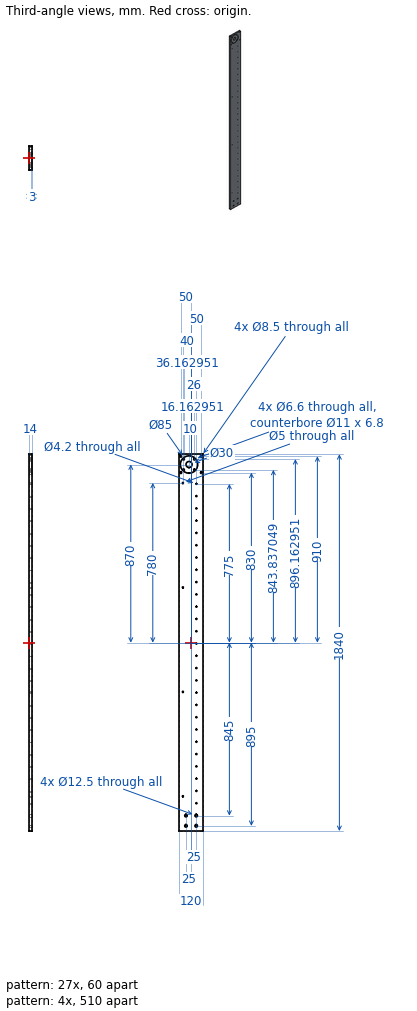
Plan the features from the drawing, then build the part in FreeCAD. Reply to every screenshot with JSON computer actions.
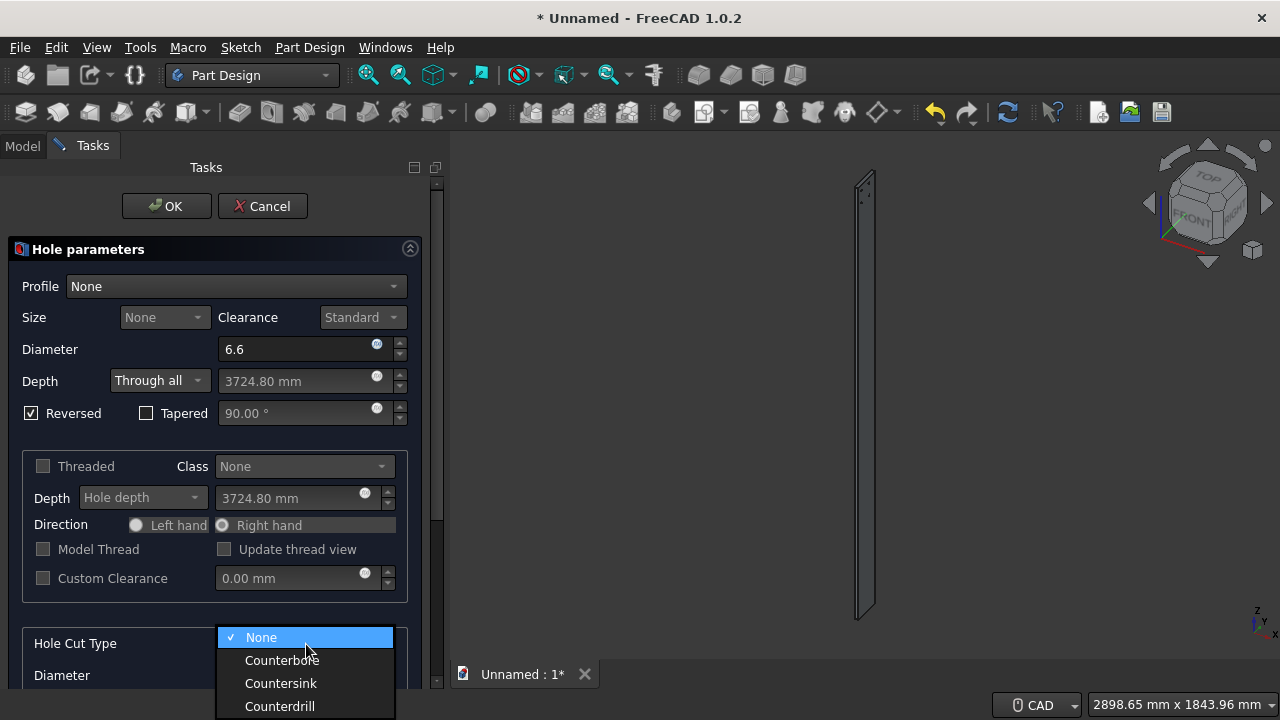
{"action": "left_click", "coordinate": [304, 660]}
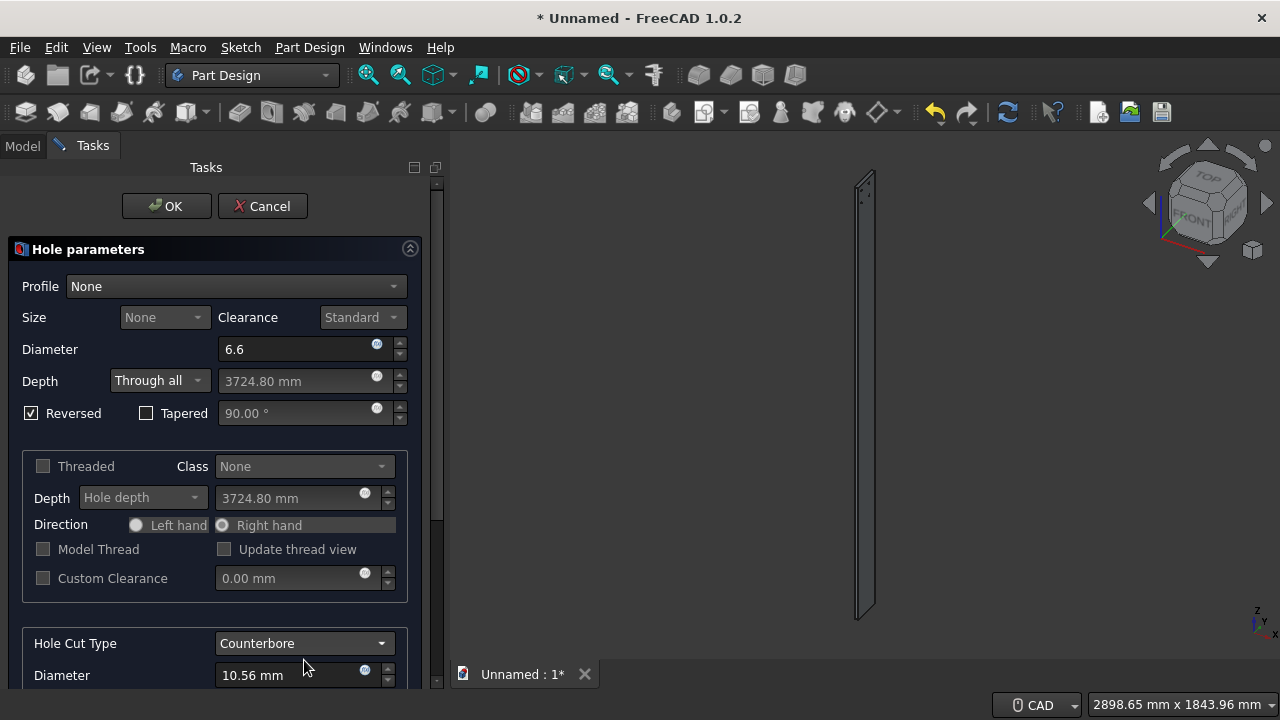
{"action": "triple_click", "coordinate": [298, 675]}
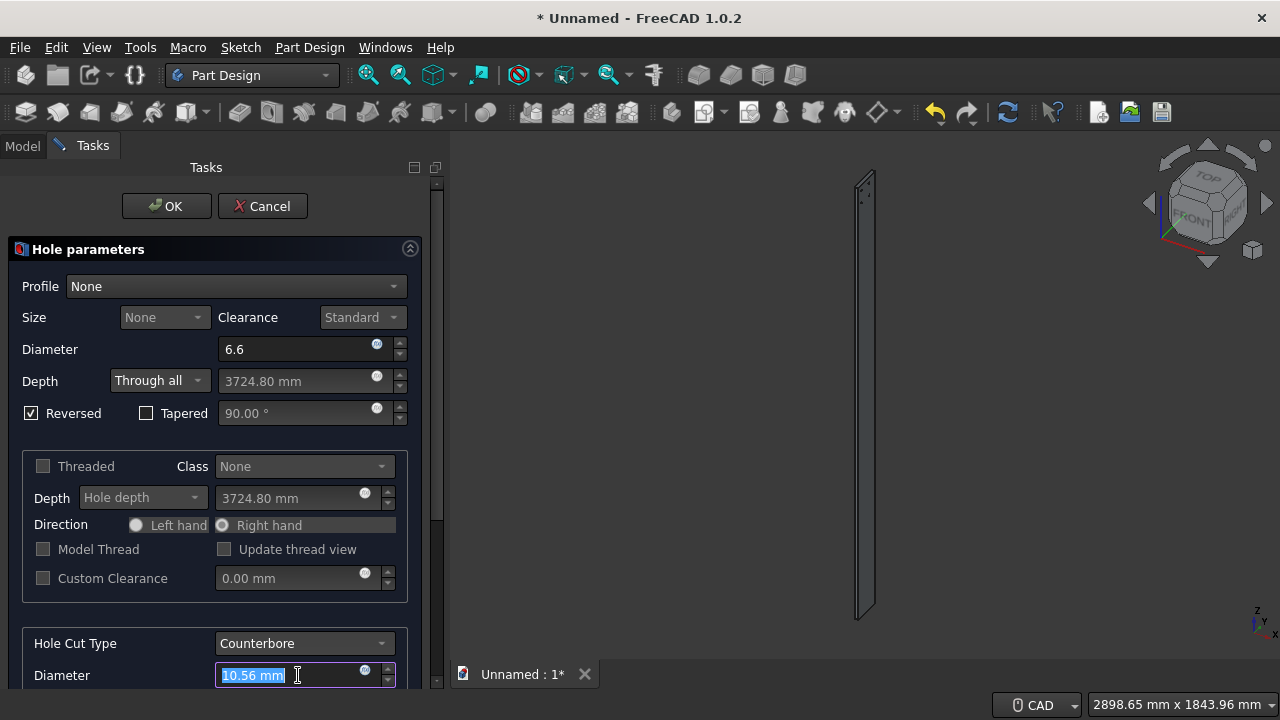
{"action": "type", "text": "11"}
{"action": "key", "text": "Tab"}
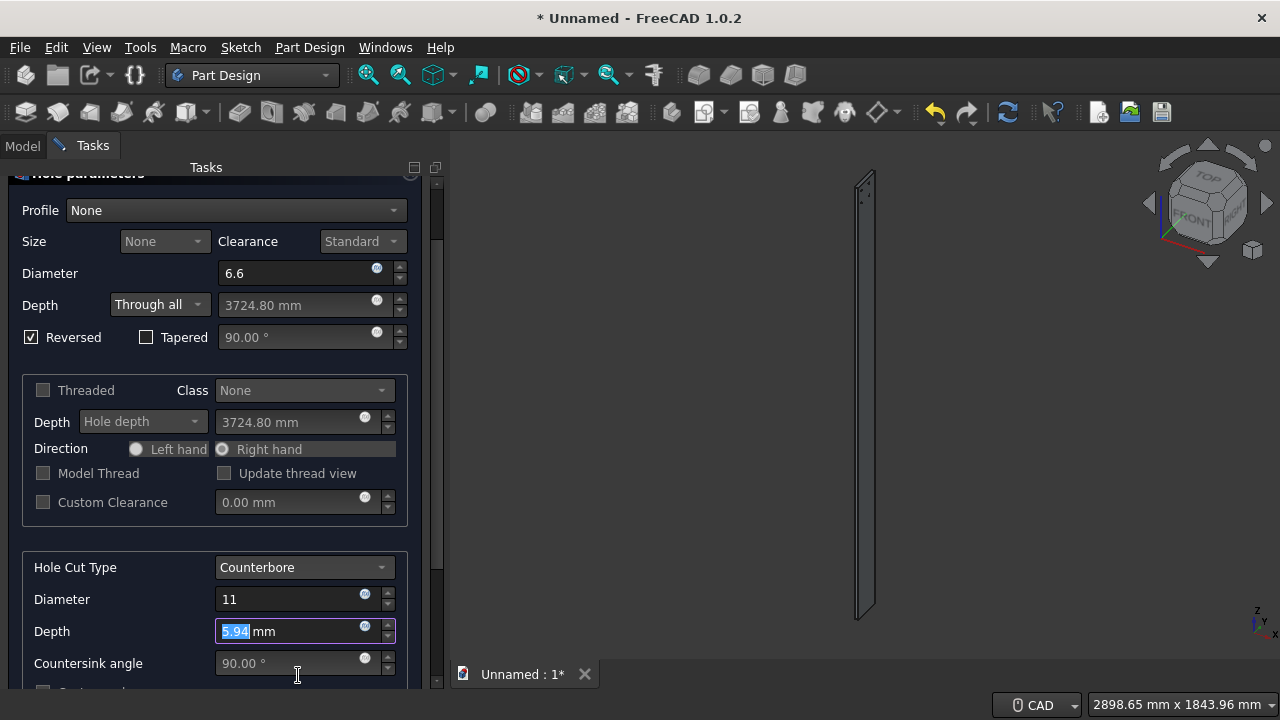
{"action": "type", "text": "6.8"}
{"action": "key", "text": "Tab"}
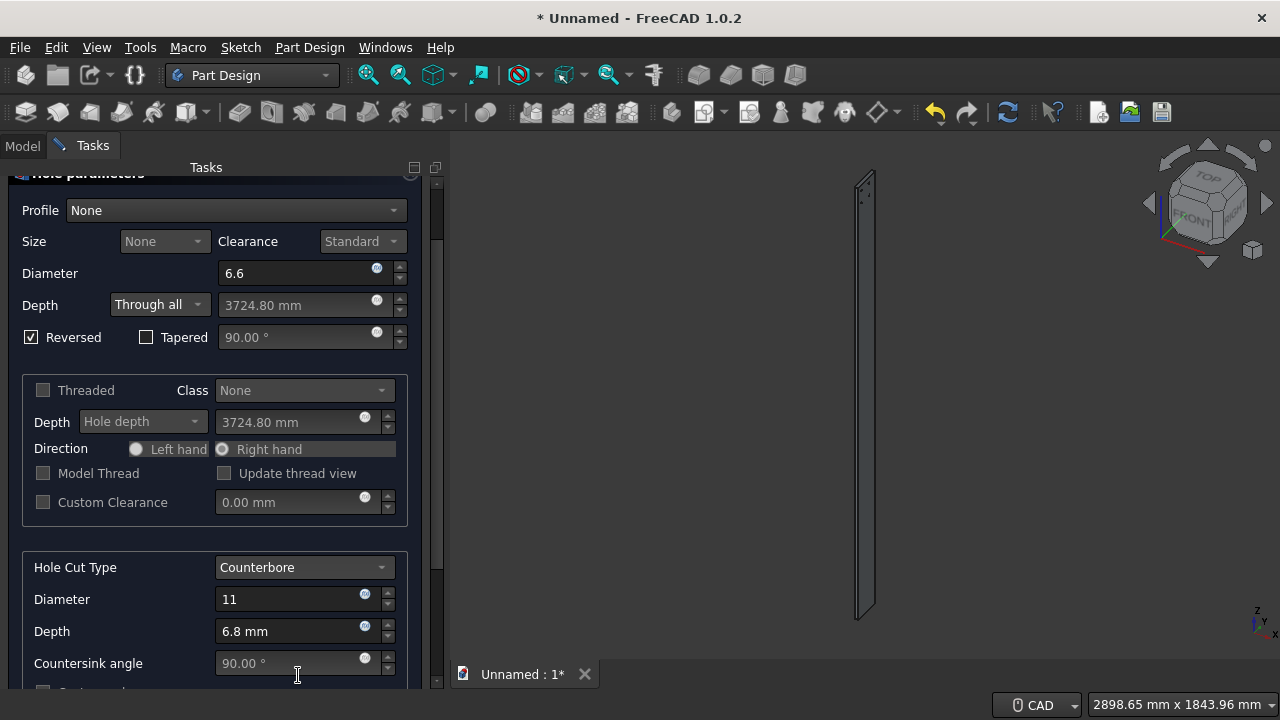
{"action": "scroll", "coordinate": [437, 432], "scroll_direction": "up", "scroll_amount": 3}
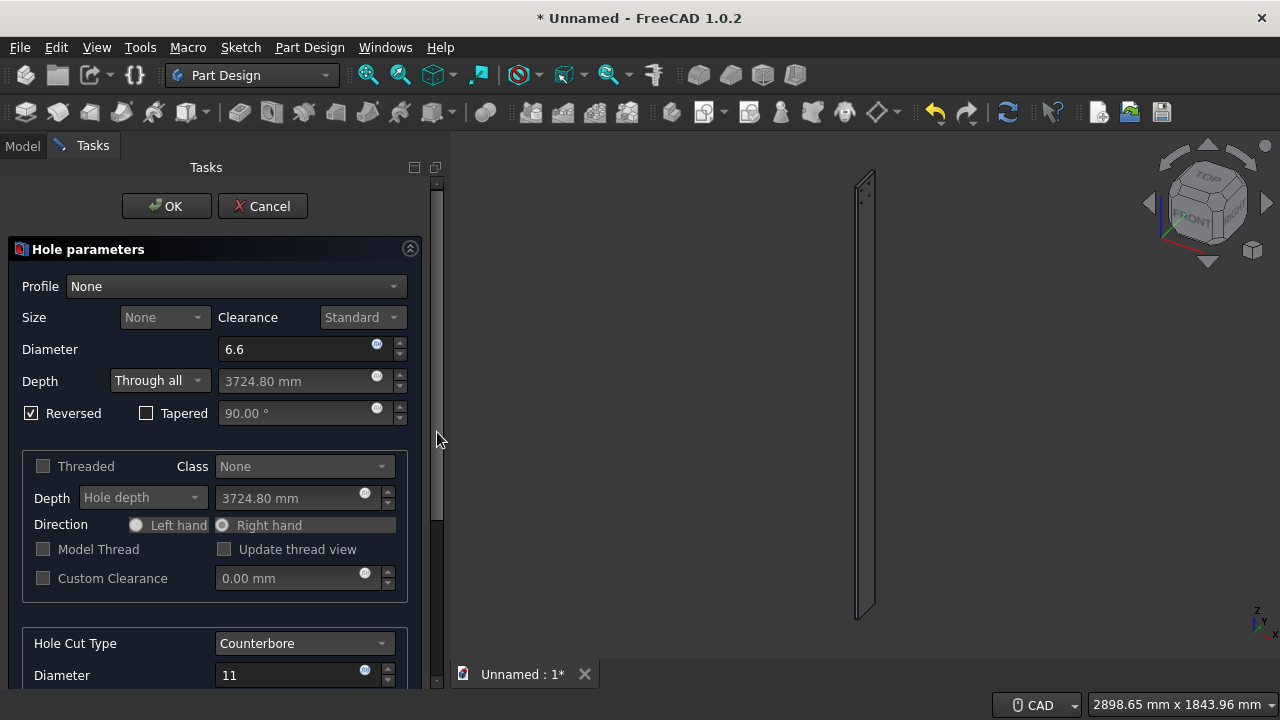
{"action": "left_click", "coordinate": [167, 206]}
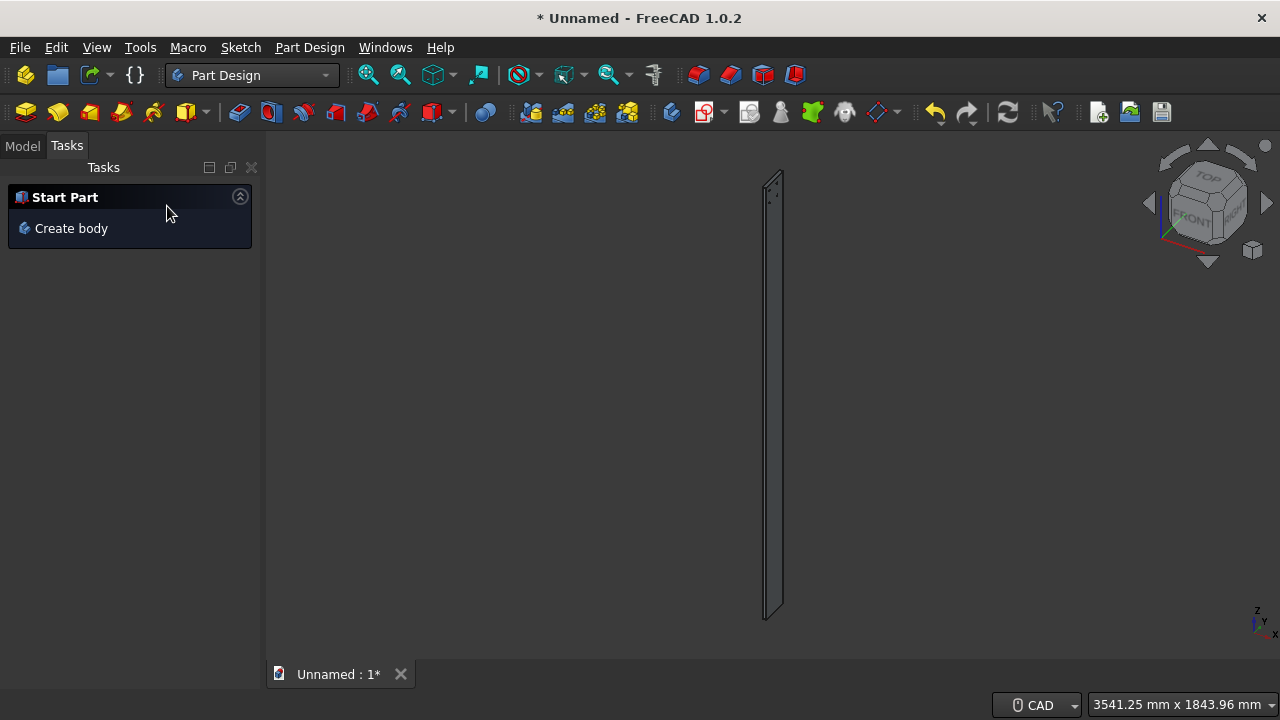
{"action": "left_click", "coordinate": [775, 456]}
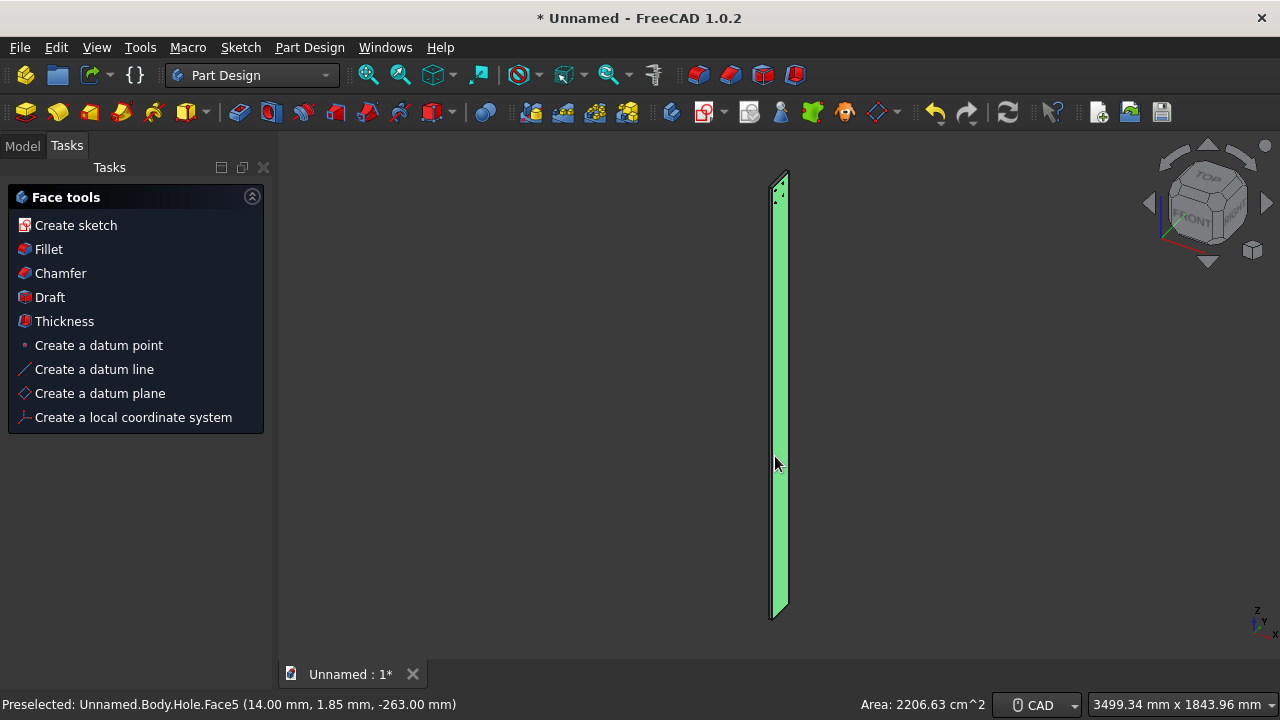
{"action": "left_click", "coordinate": [704, 112]}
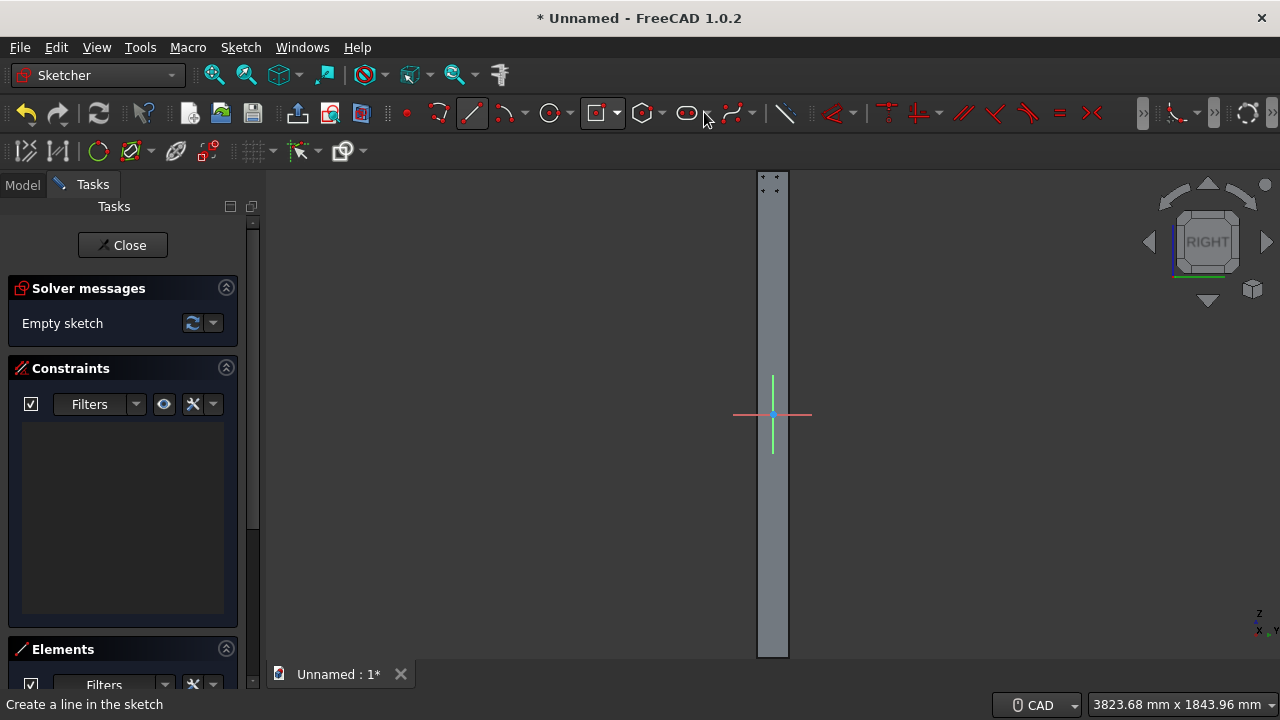
{"action": "scroll", "coordinate": [784, 198], "scroll_direction": "up", "scroll_amount": 15}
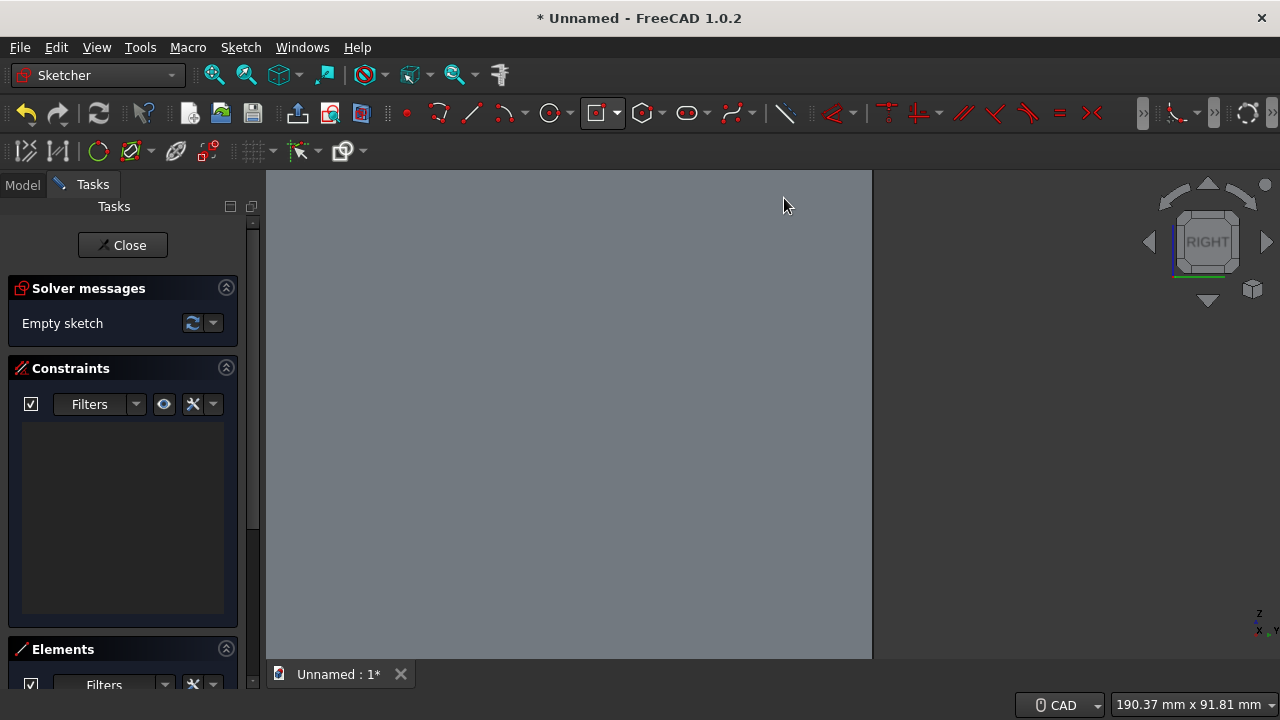
{"action": "scroll", "coordinate": [691, 418], "scroll_direction": "up", "scroll_amount": 13}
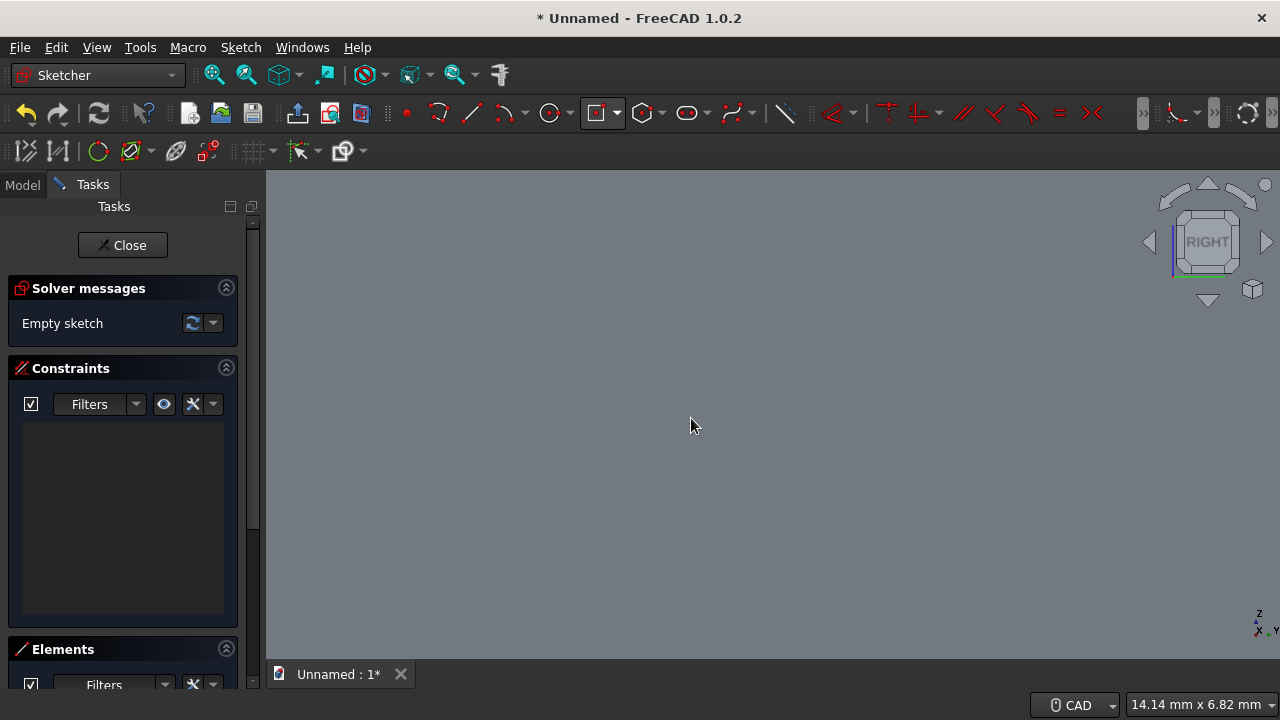
{"action": "left_click", "coordinate": [550, 114]}